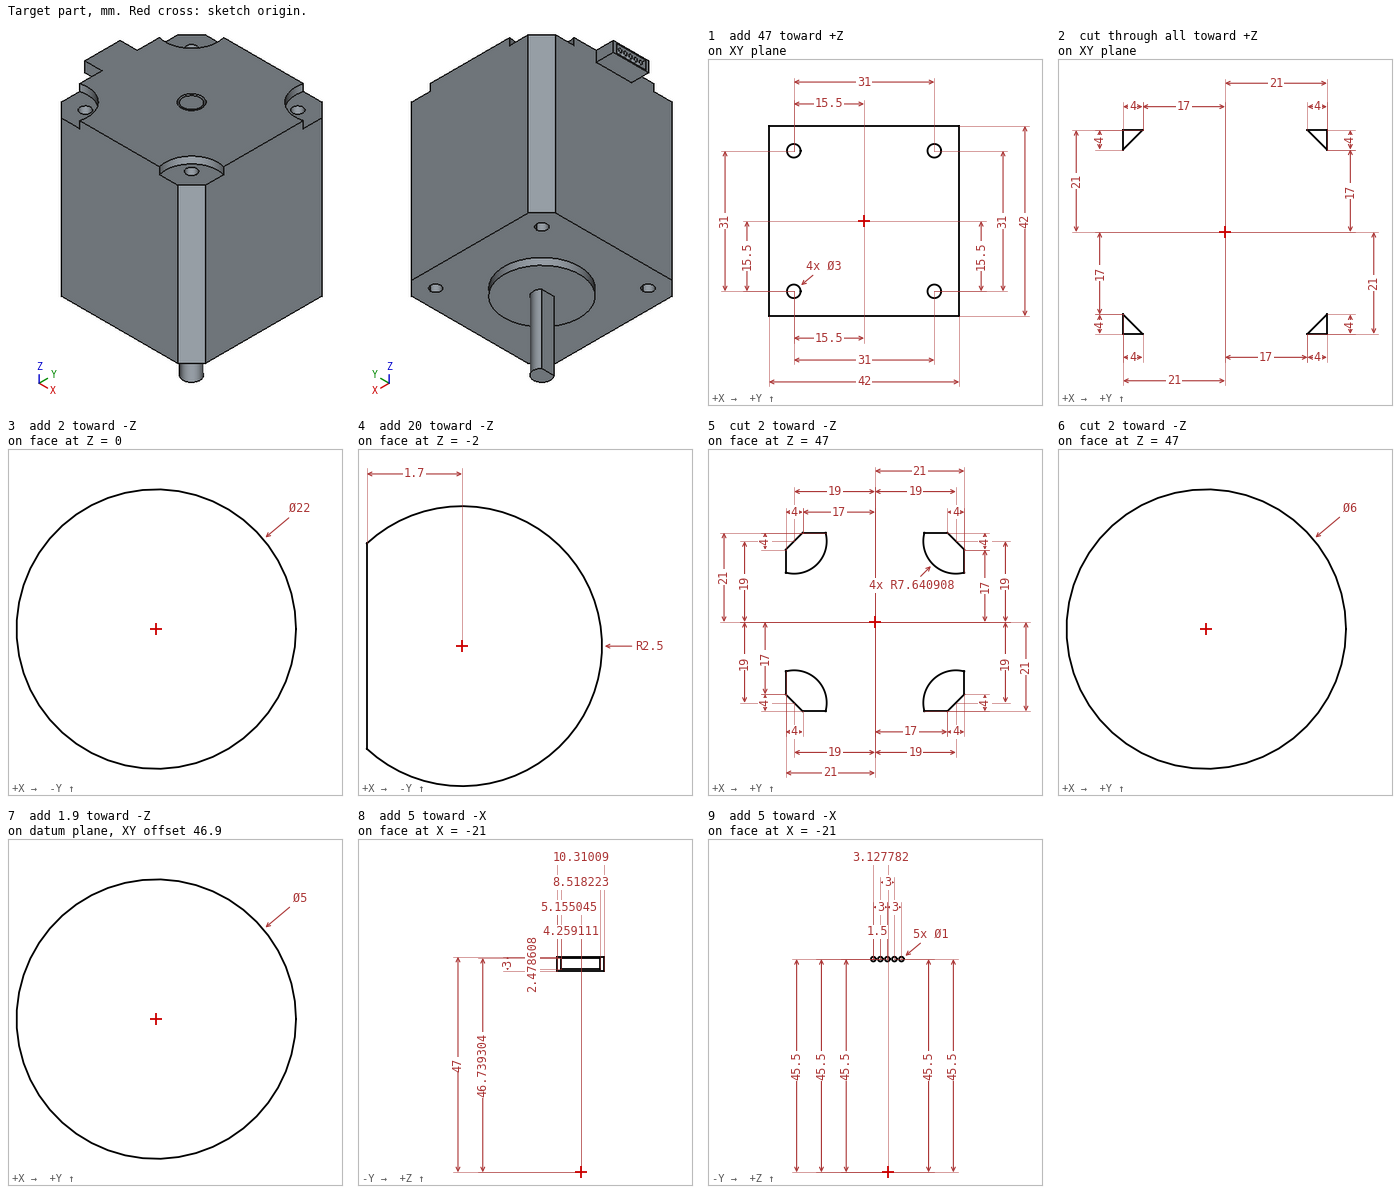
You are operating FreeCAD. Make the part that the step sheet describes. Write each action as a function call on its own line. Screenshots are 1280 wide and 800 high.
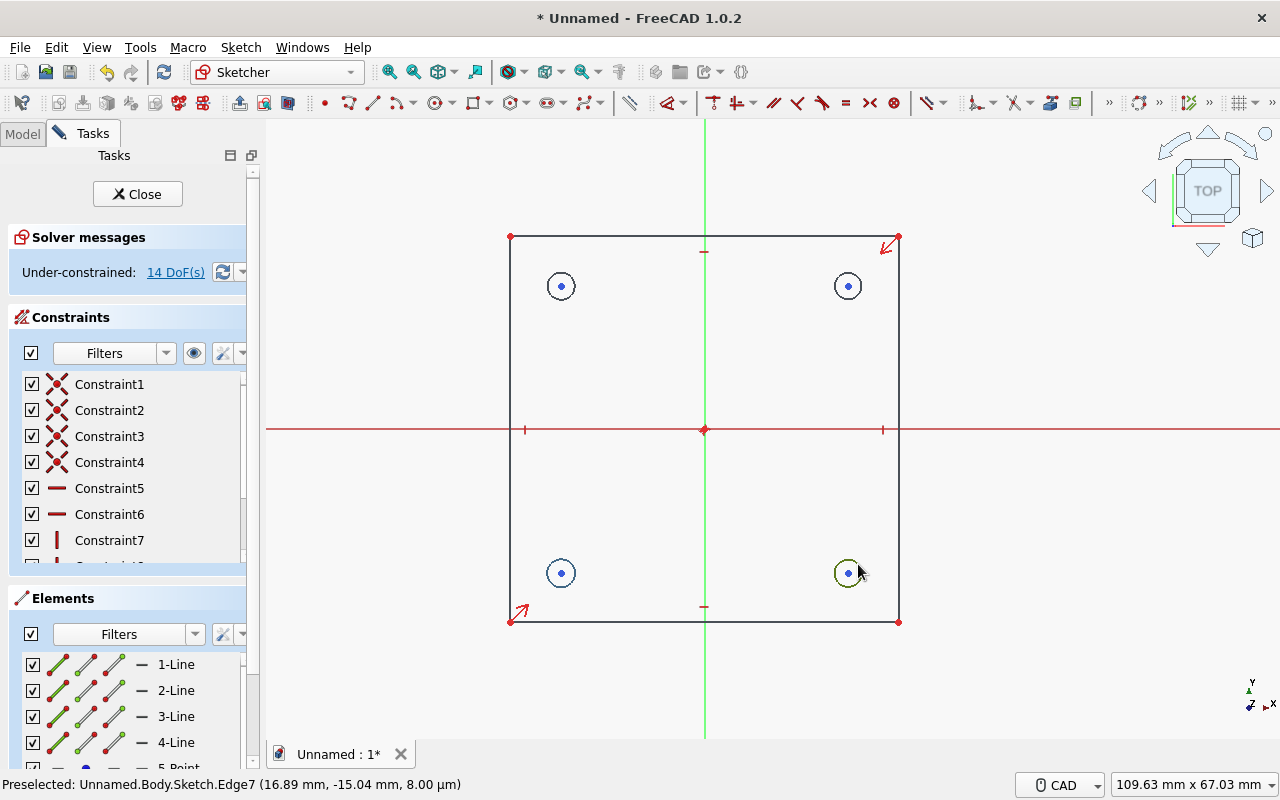
click(571, 276)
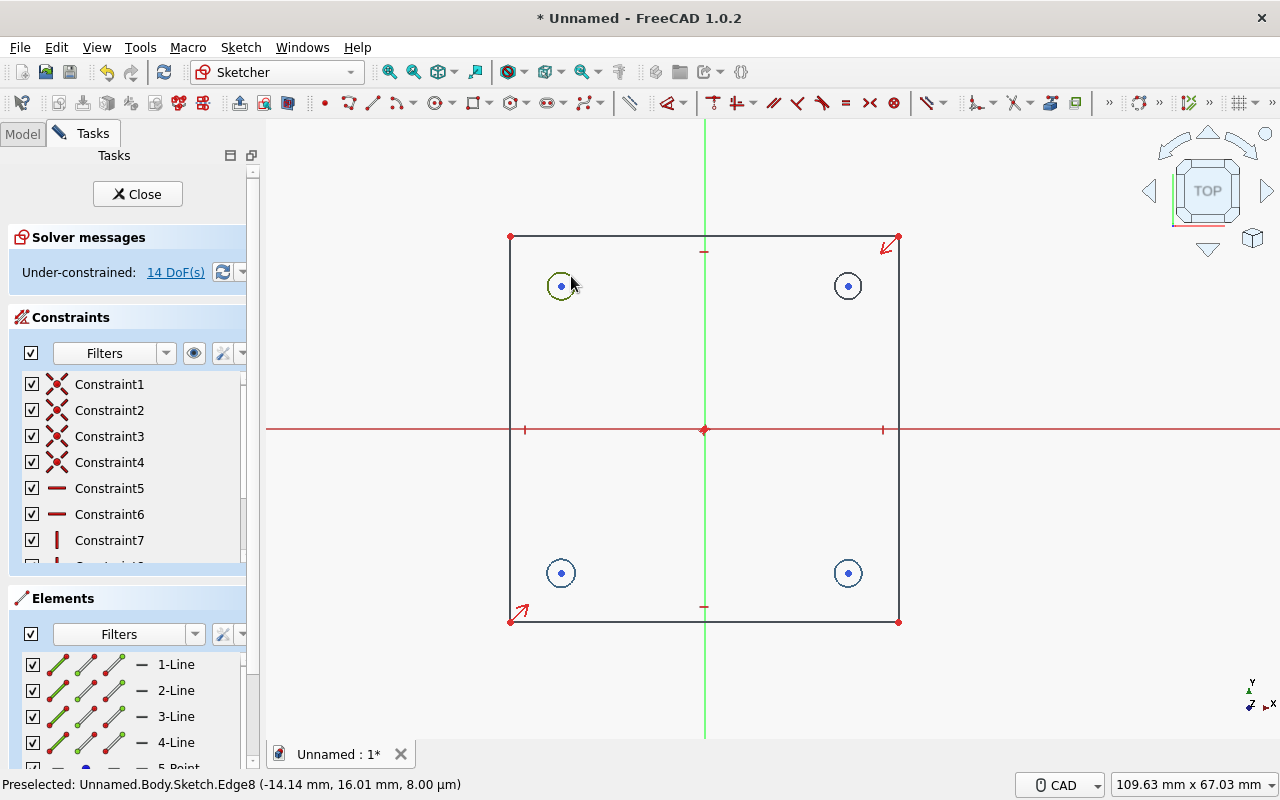
click(857, 277)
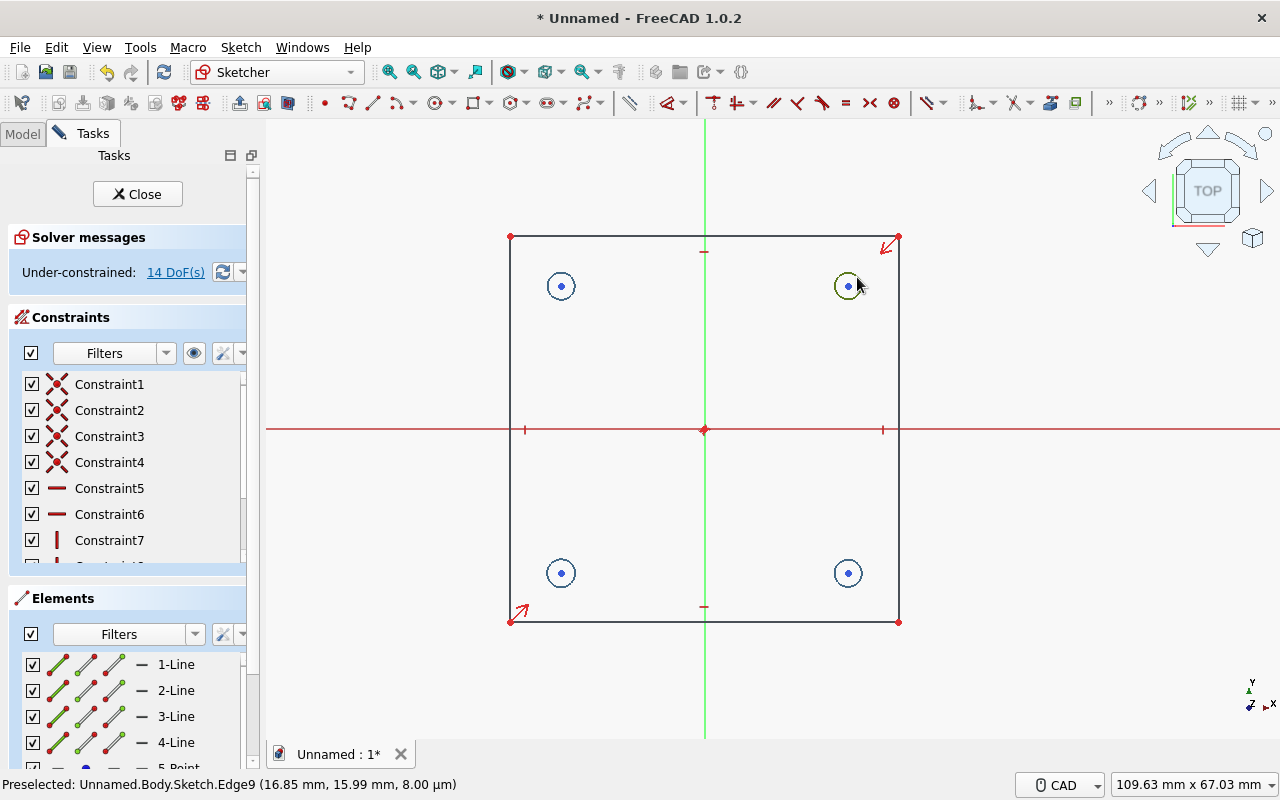
click(846, 104)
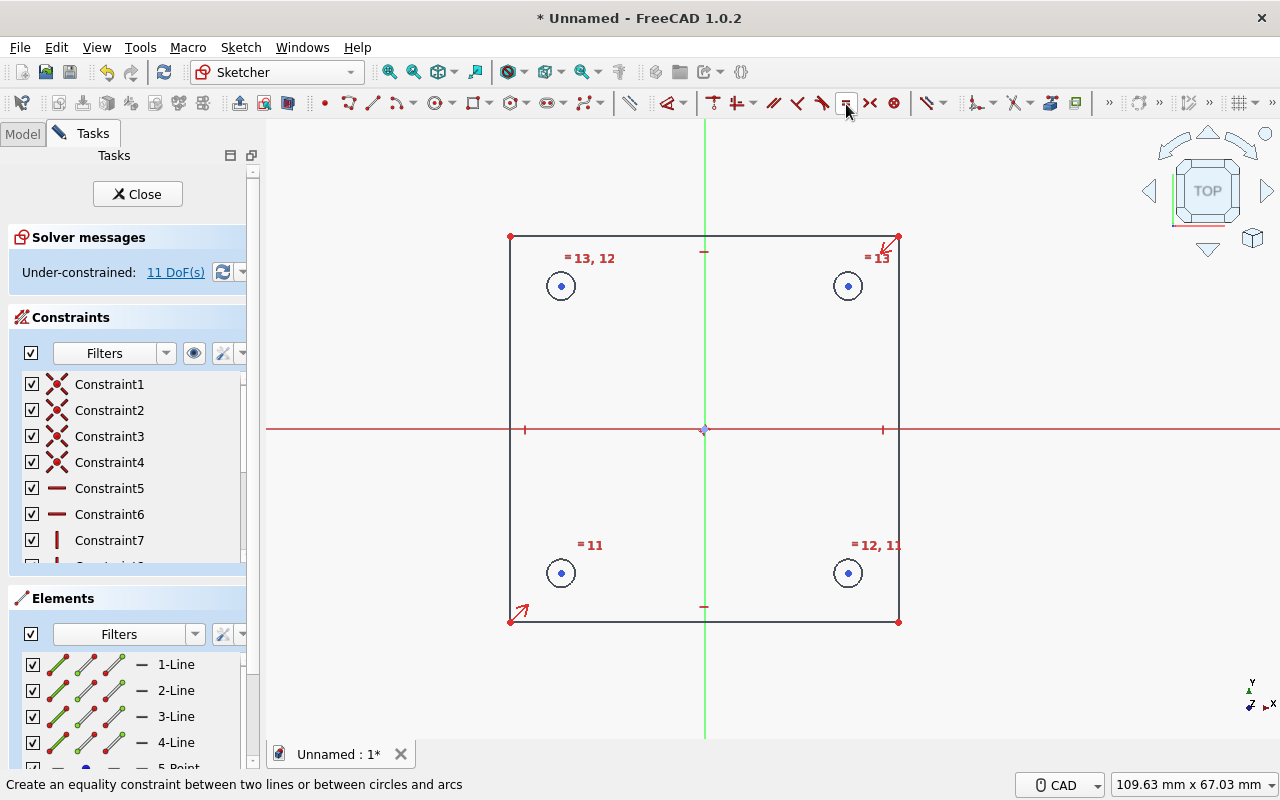
scroll(571, 563, up, 2)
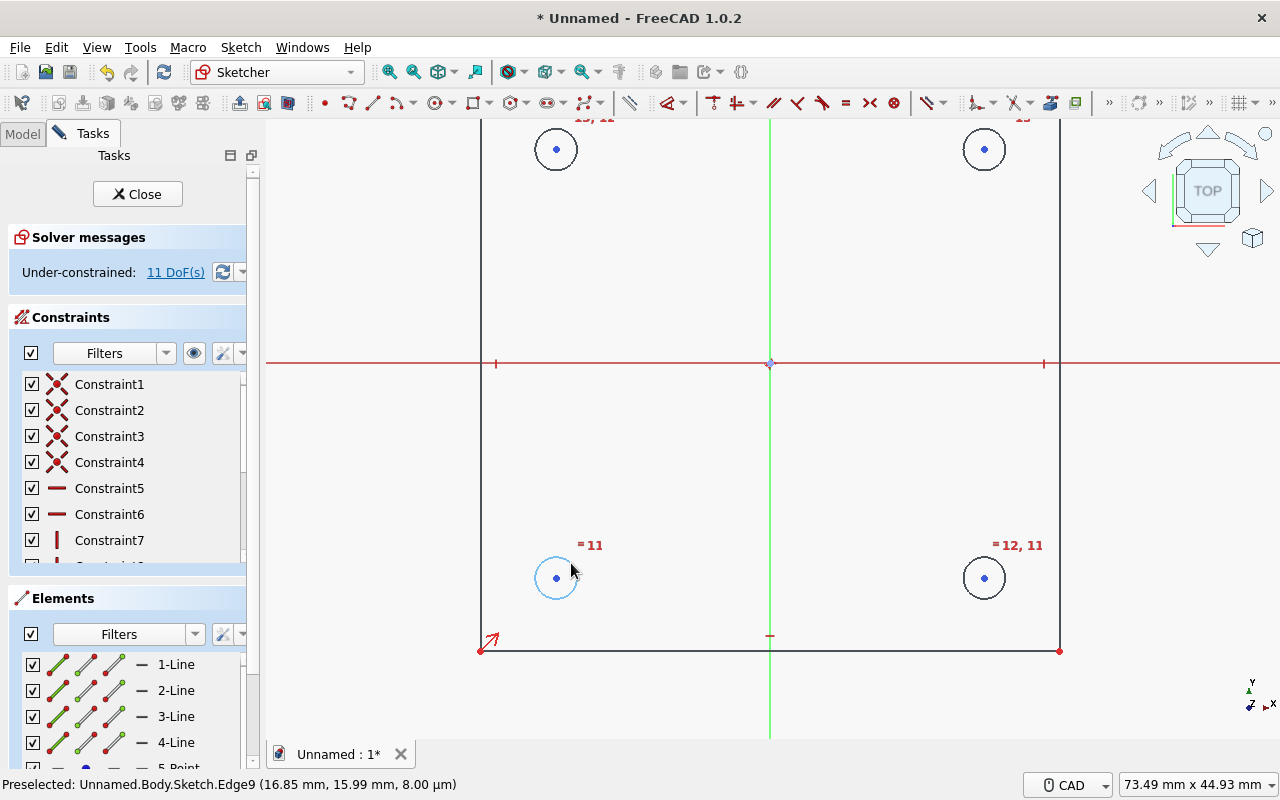
click(571, 563)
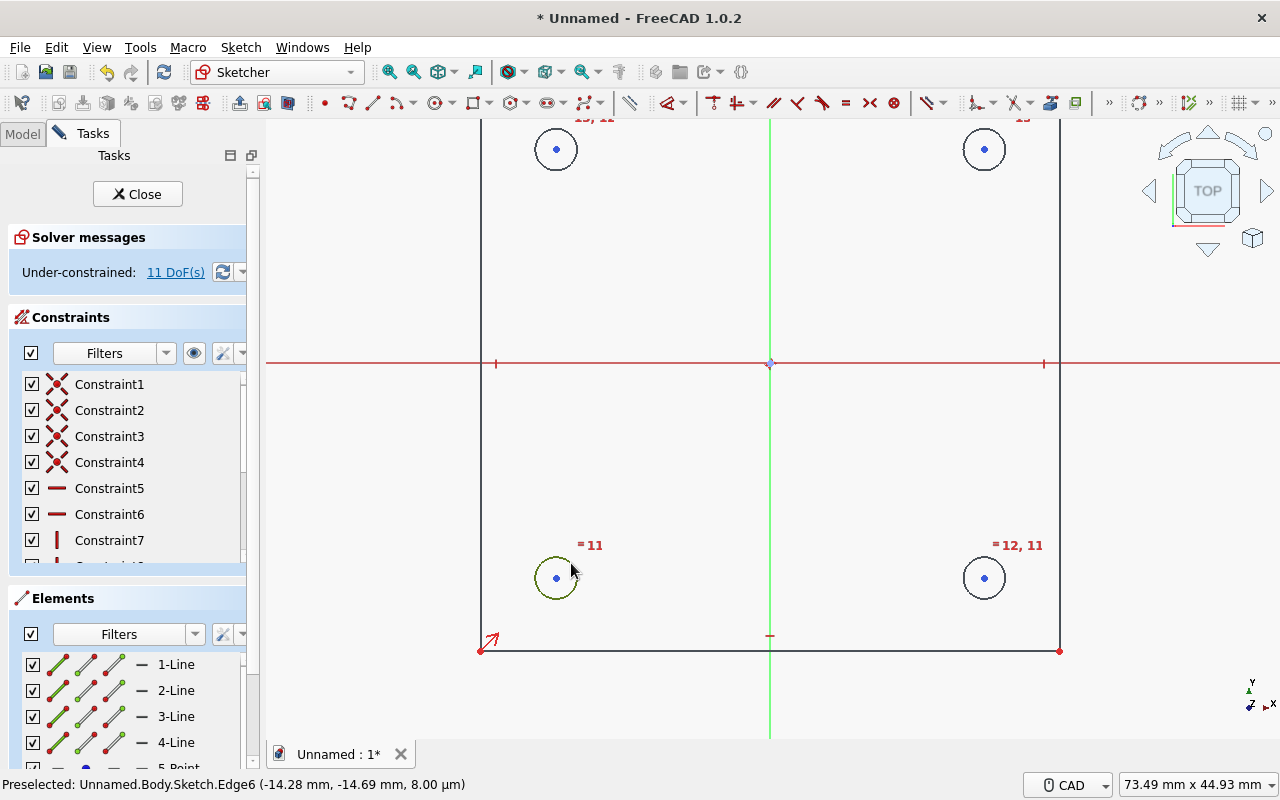
click(686, 104)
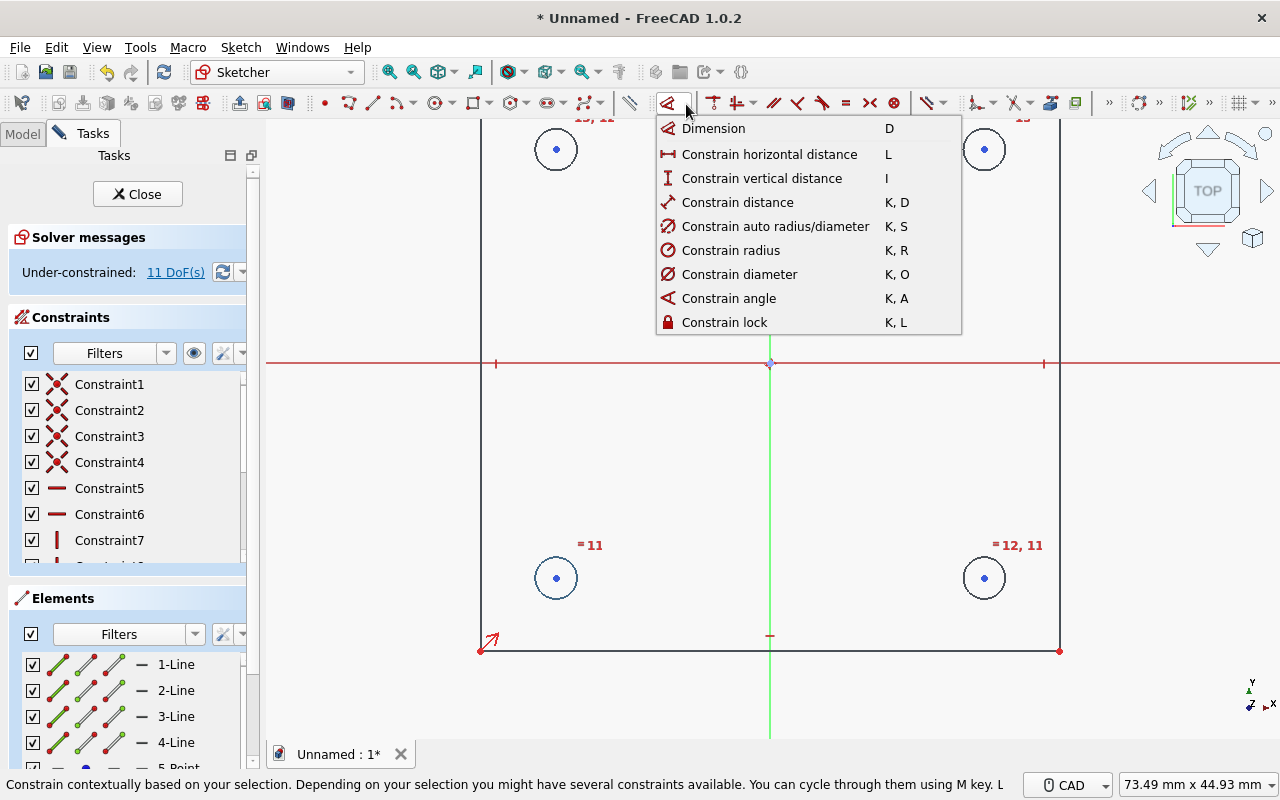
click(809, 274)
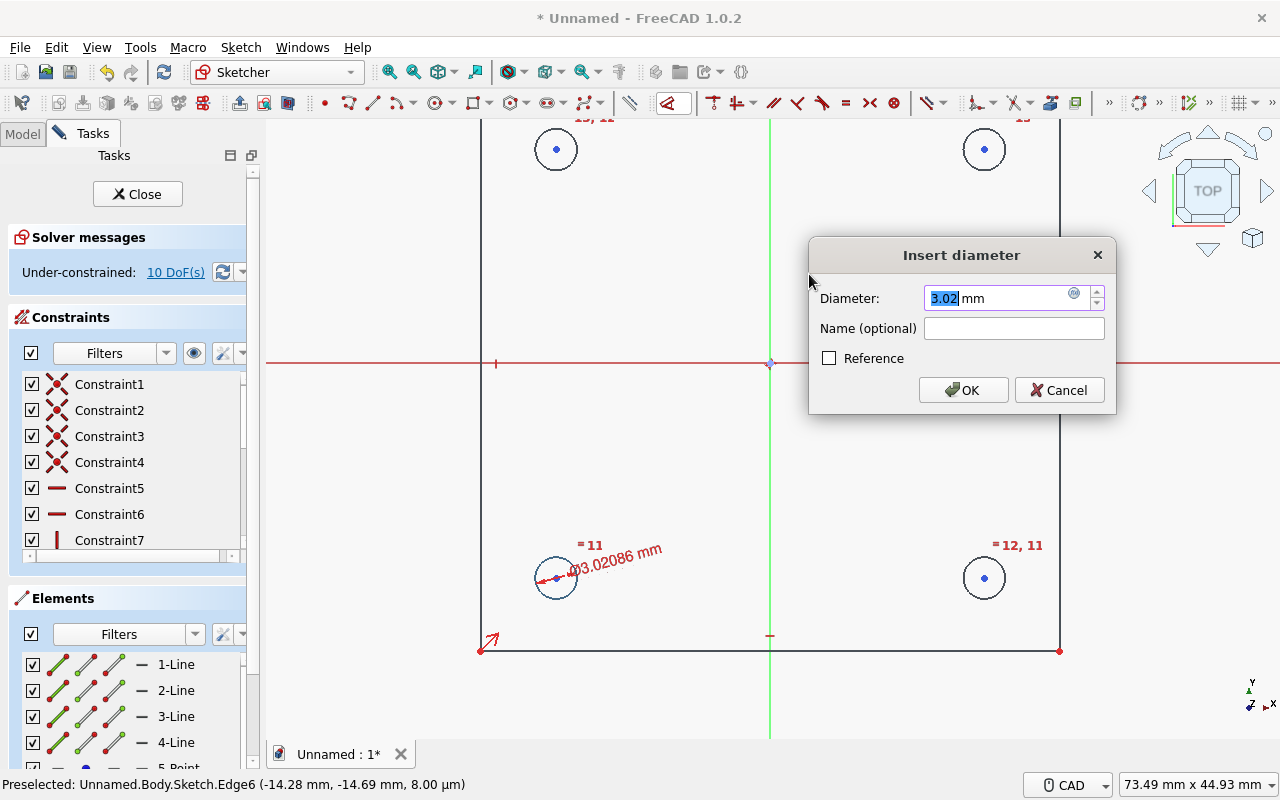
text(3)
key(Return)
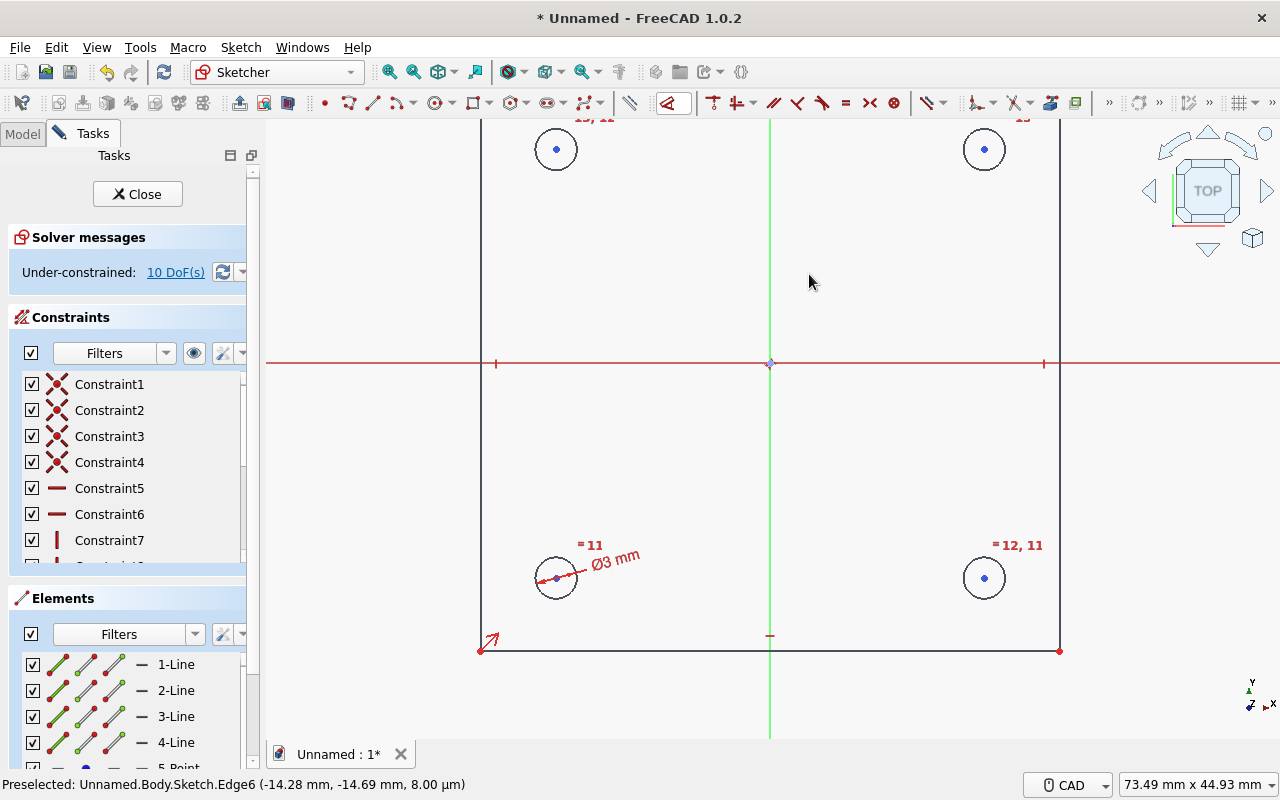
click(654, 651)